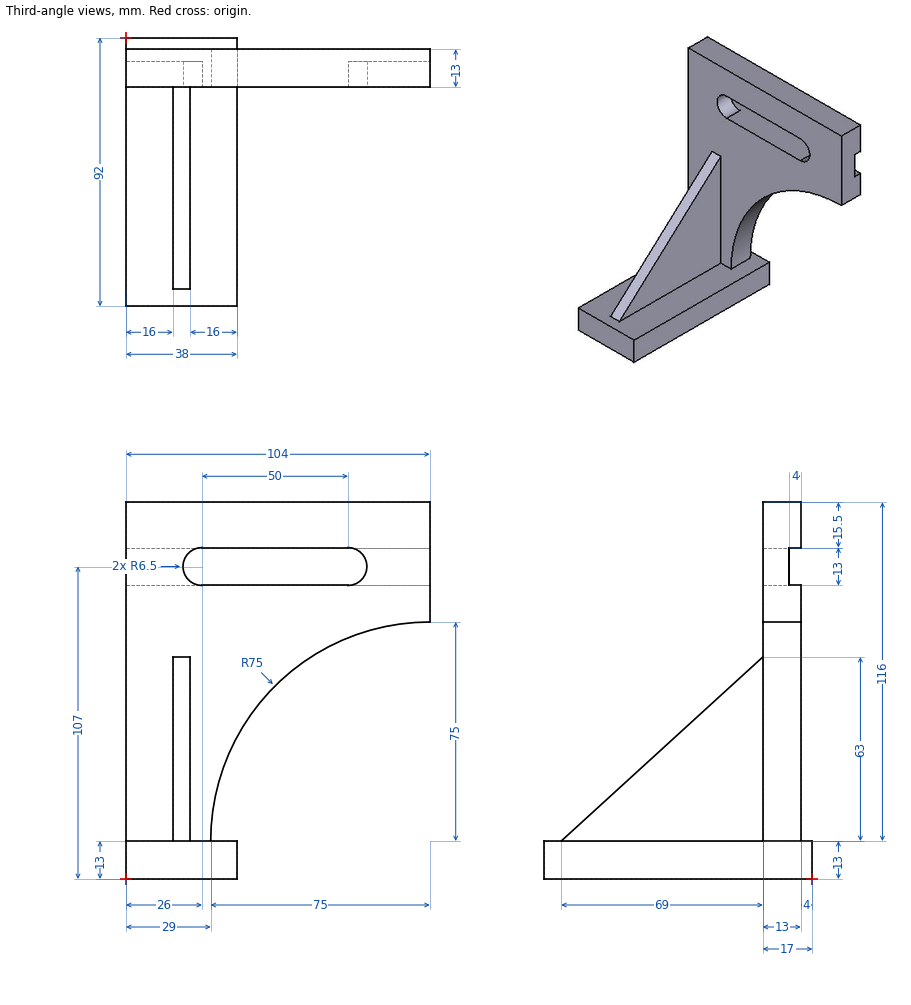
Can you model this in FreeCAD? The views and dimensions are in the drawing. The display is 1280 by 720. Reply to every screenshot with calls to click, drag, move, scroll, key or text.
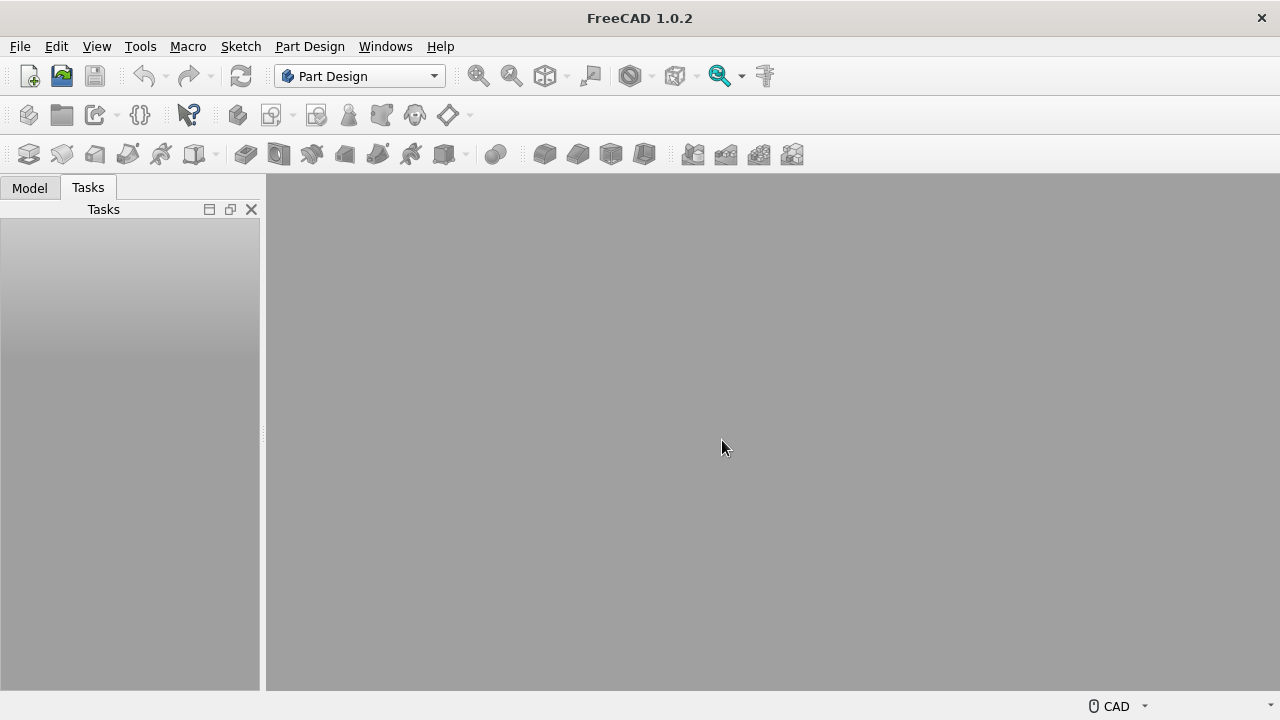
click(29, 76)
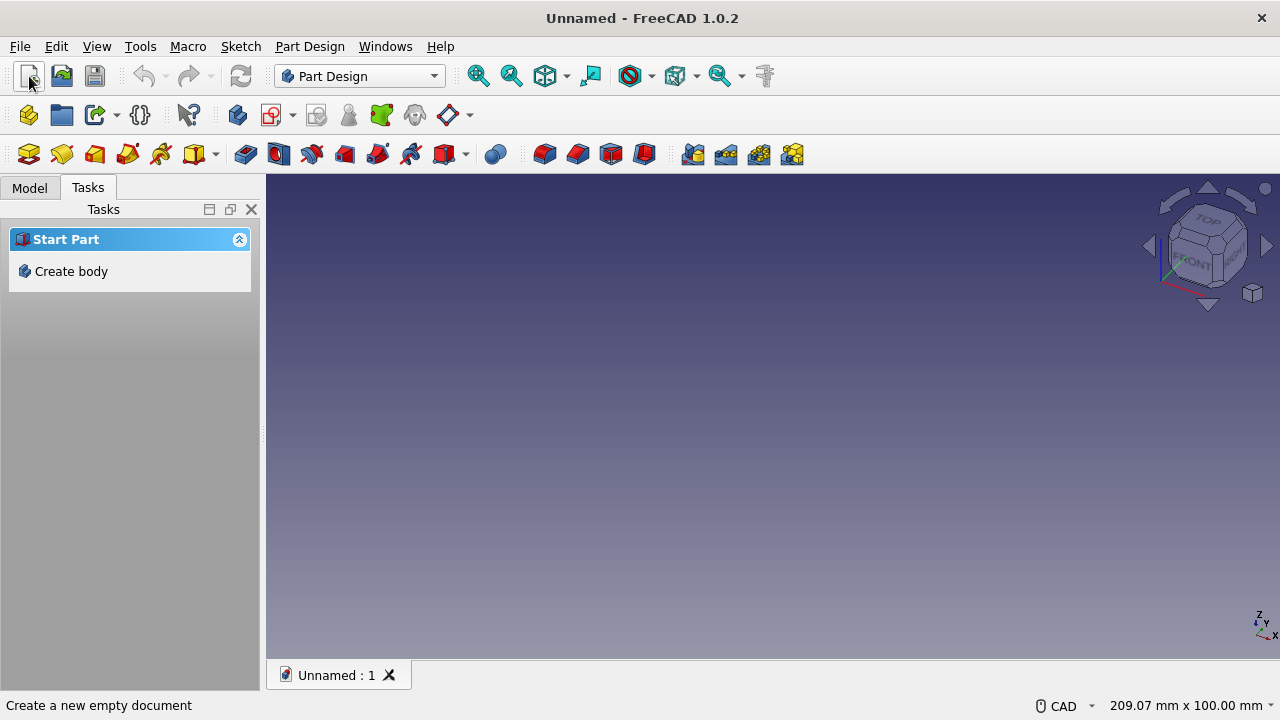
click(270, 116)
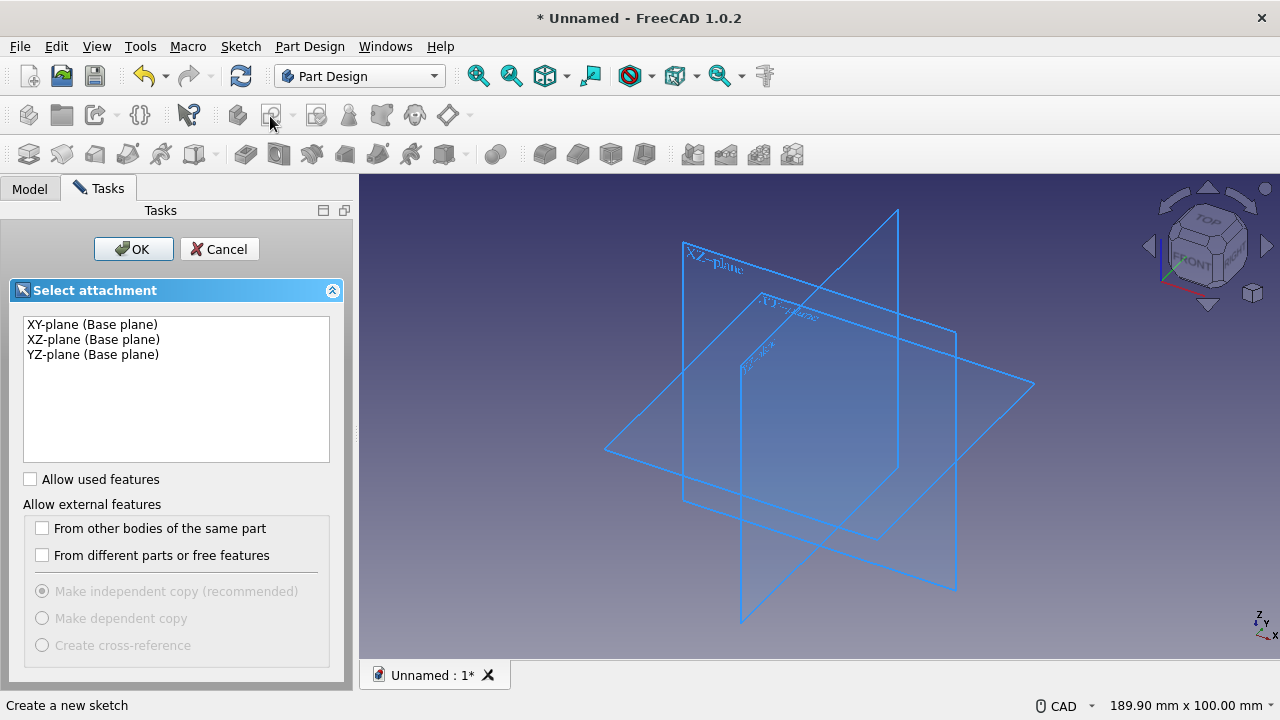
click(84, 324)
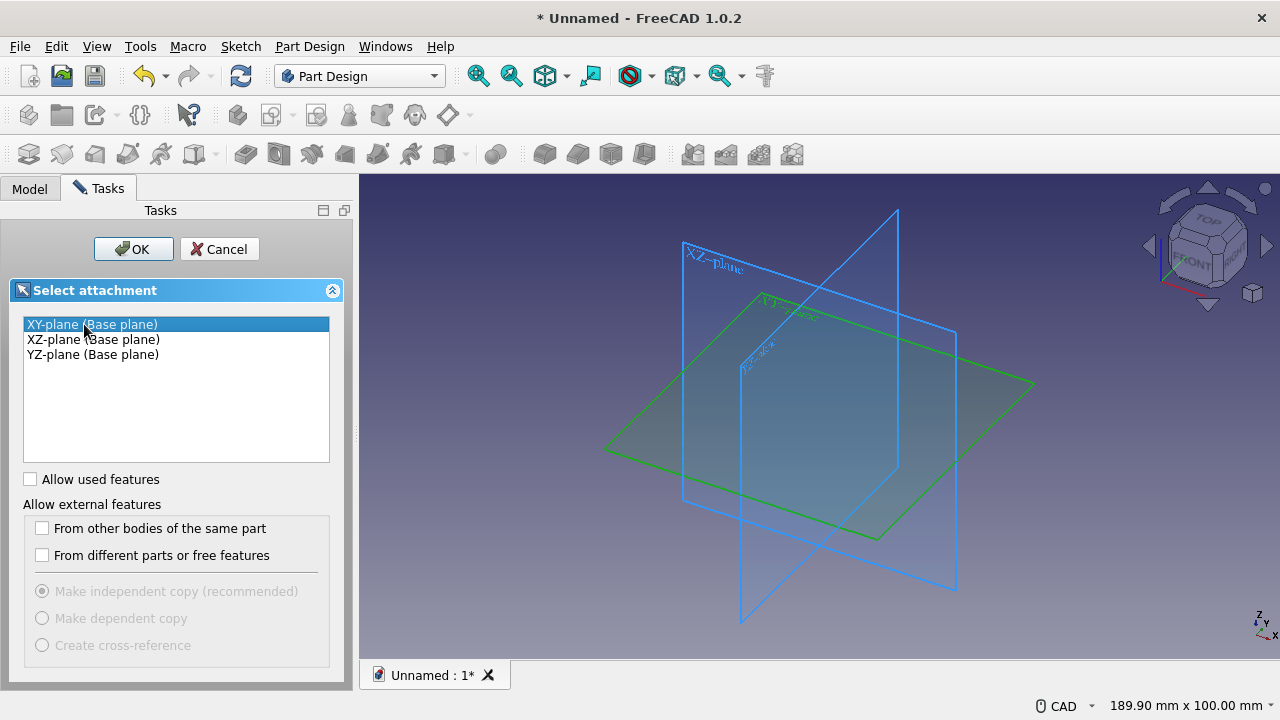
click(134, 249)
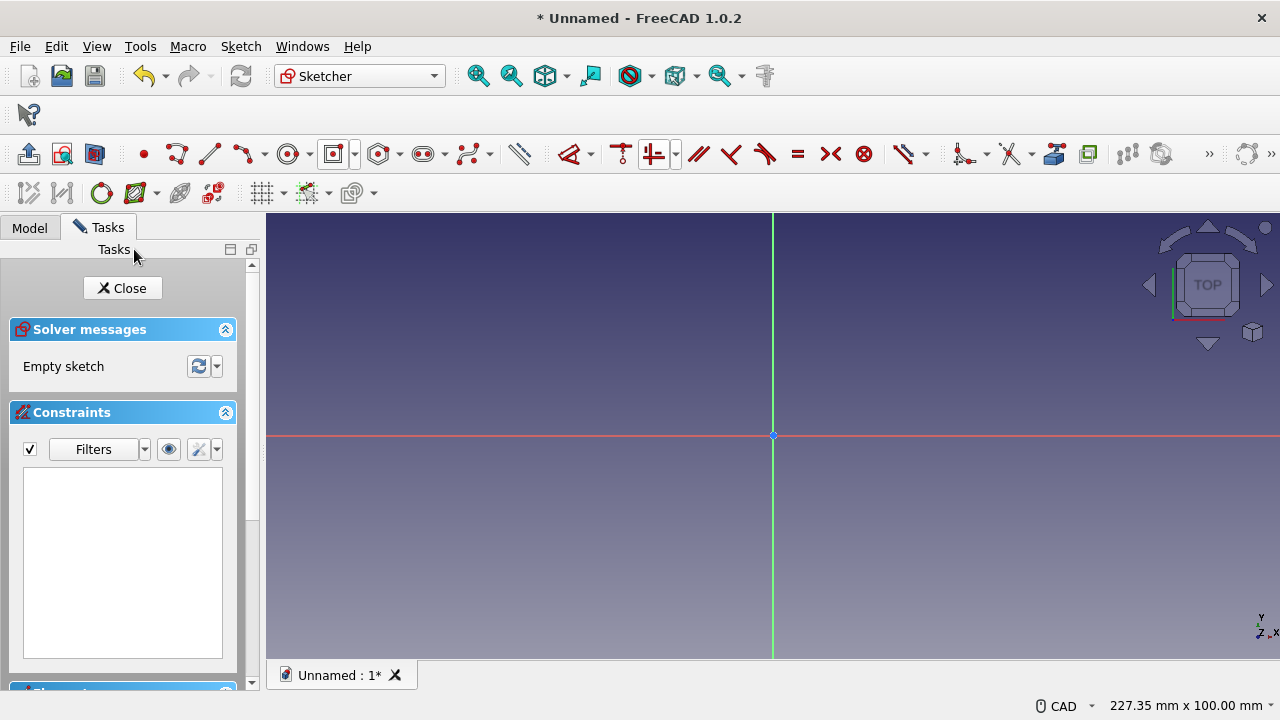
scroll(518, 241, down, 3)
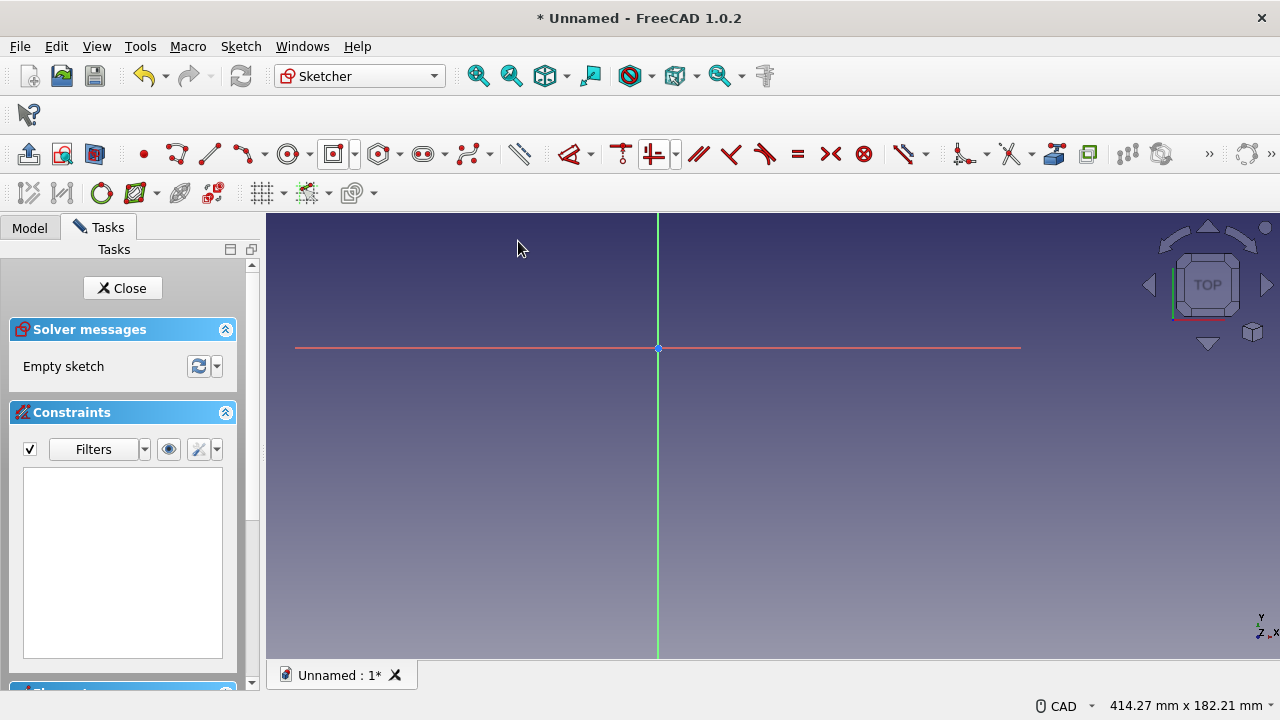
key(g)
key(r)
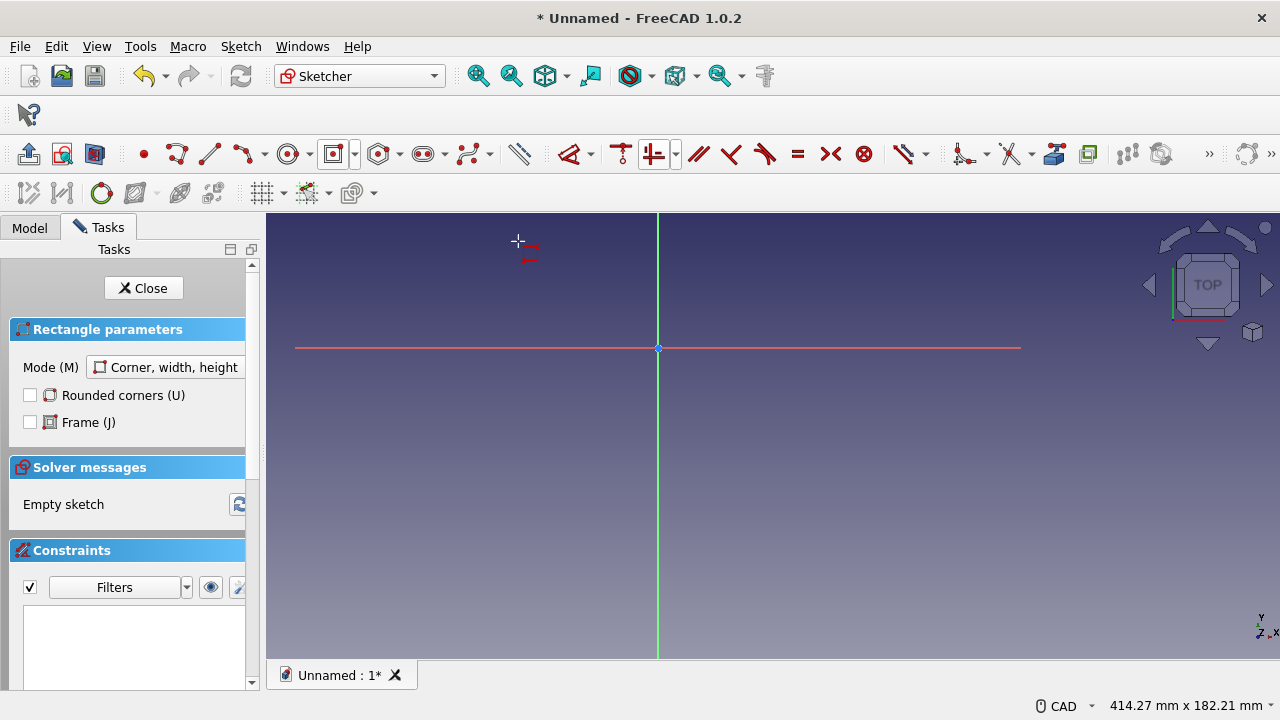
click(658, 348)
click(751, 573)
key(Escape)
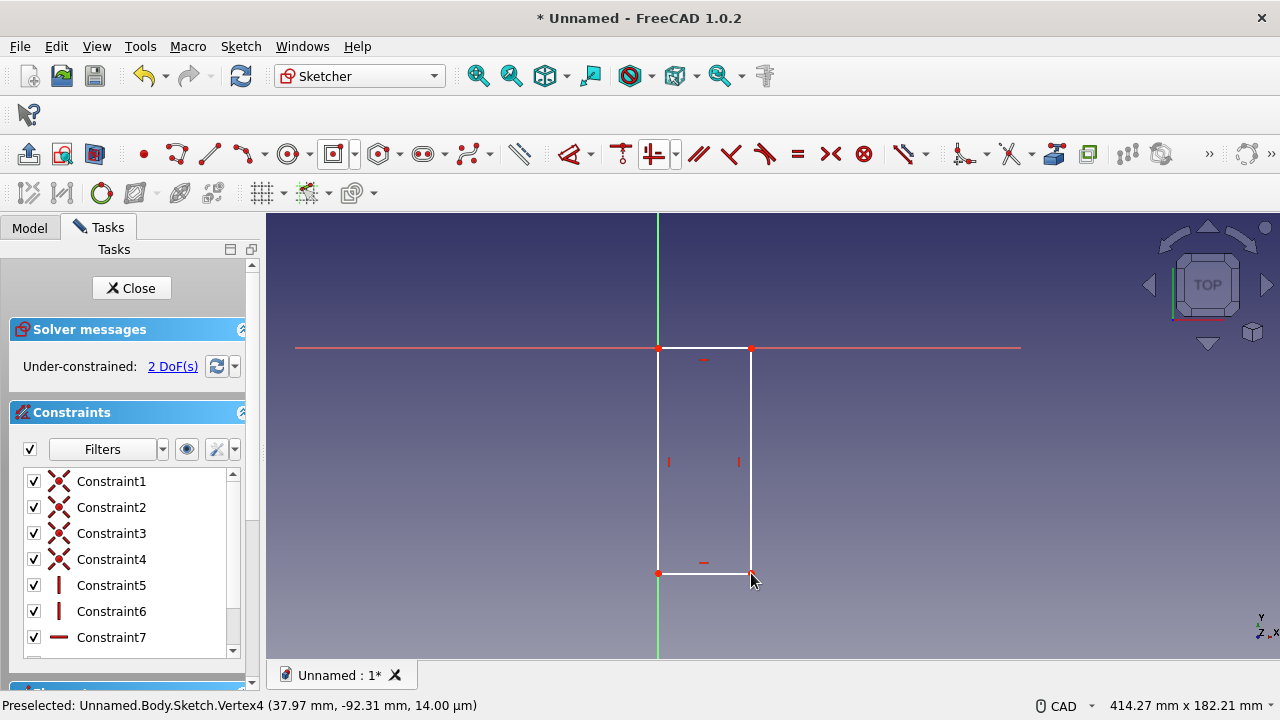
key(d)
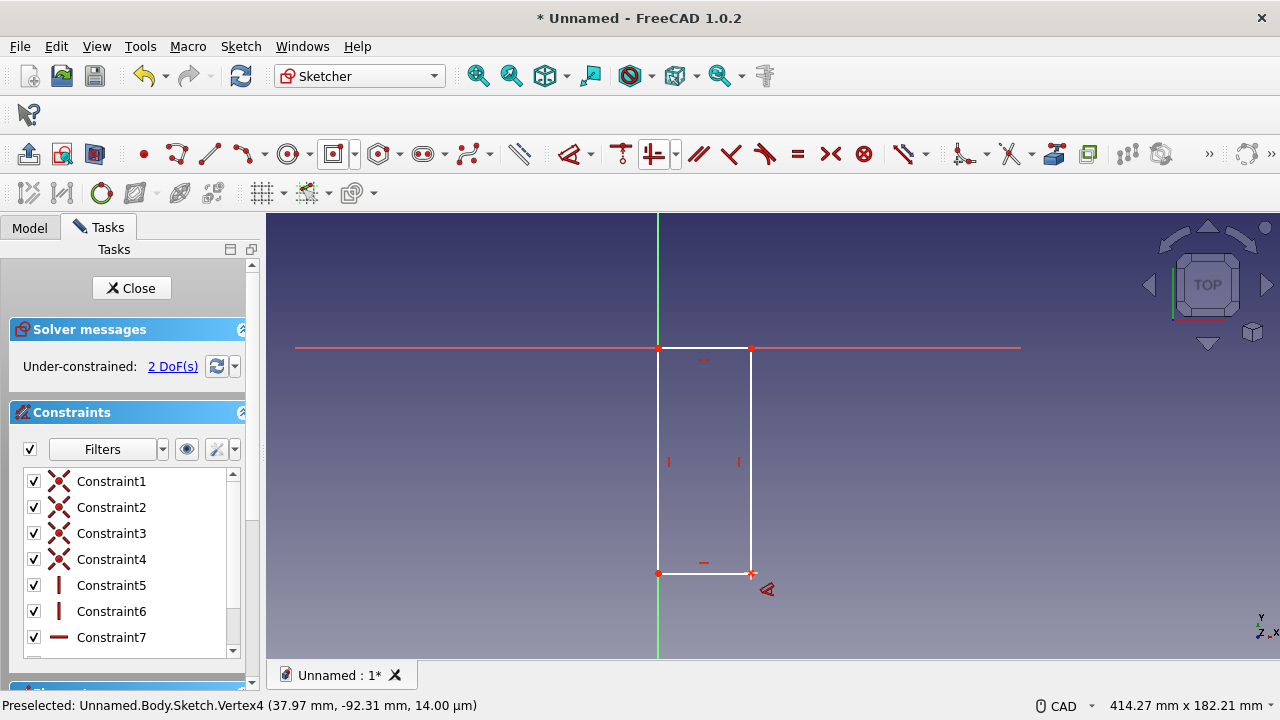
click(658, 416)
click(624, 461)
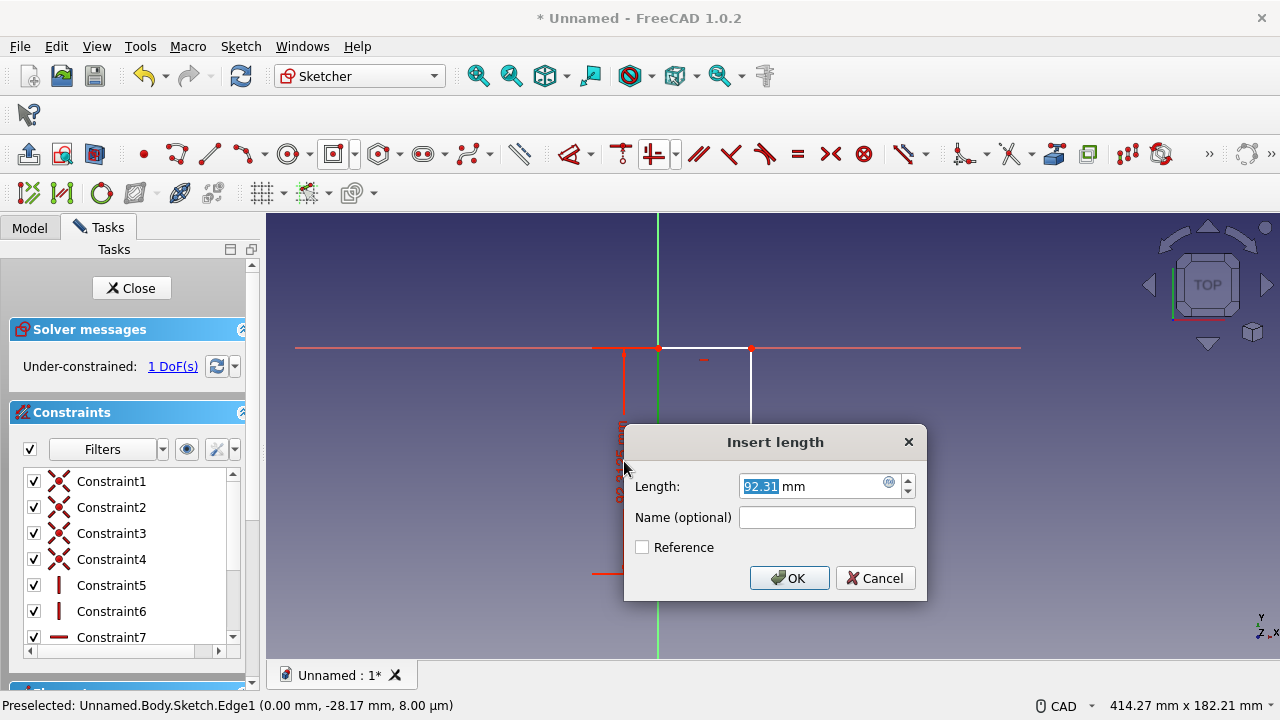
text(92)
key(Return)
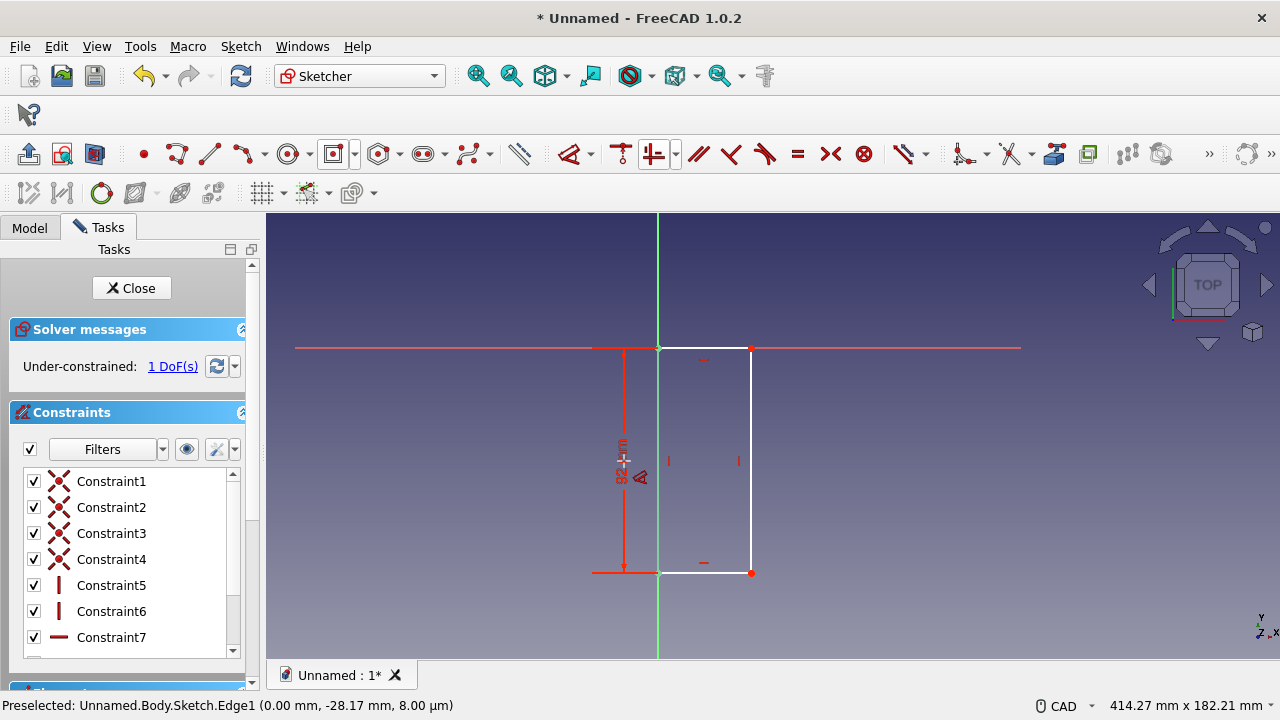
click(686, 573)
click(705, 607)